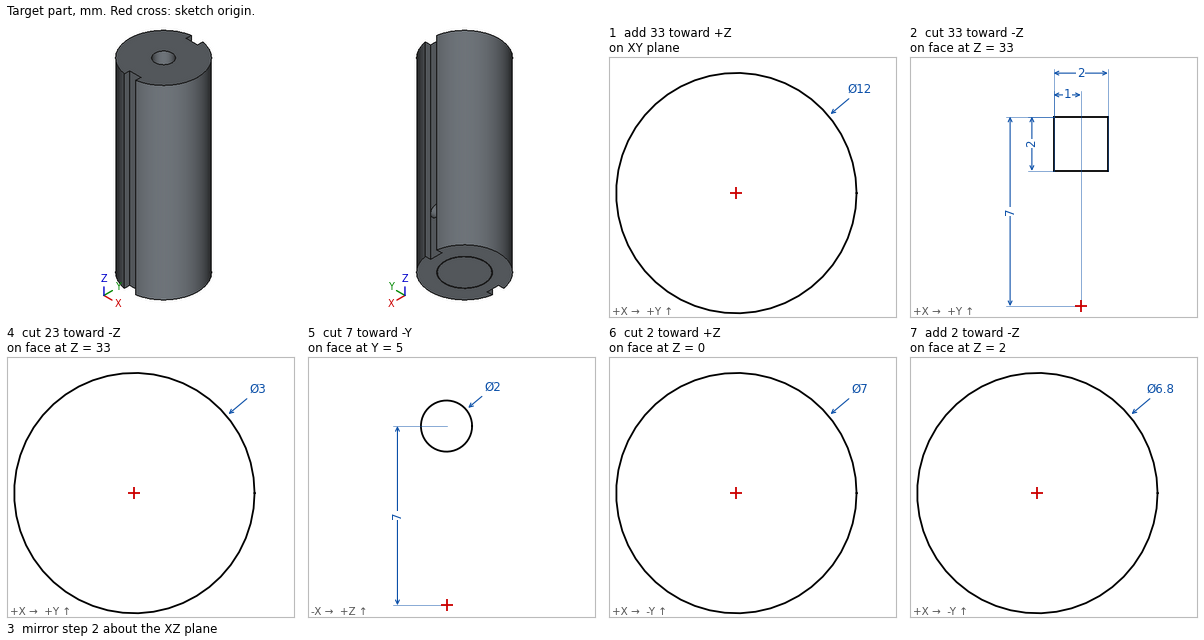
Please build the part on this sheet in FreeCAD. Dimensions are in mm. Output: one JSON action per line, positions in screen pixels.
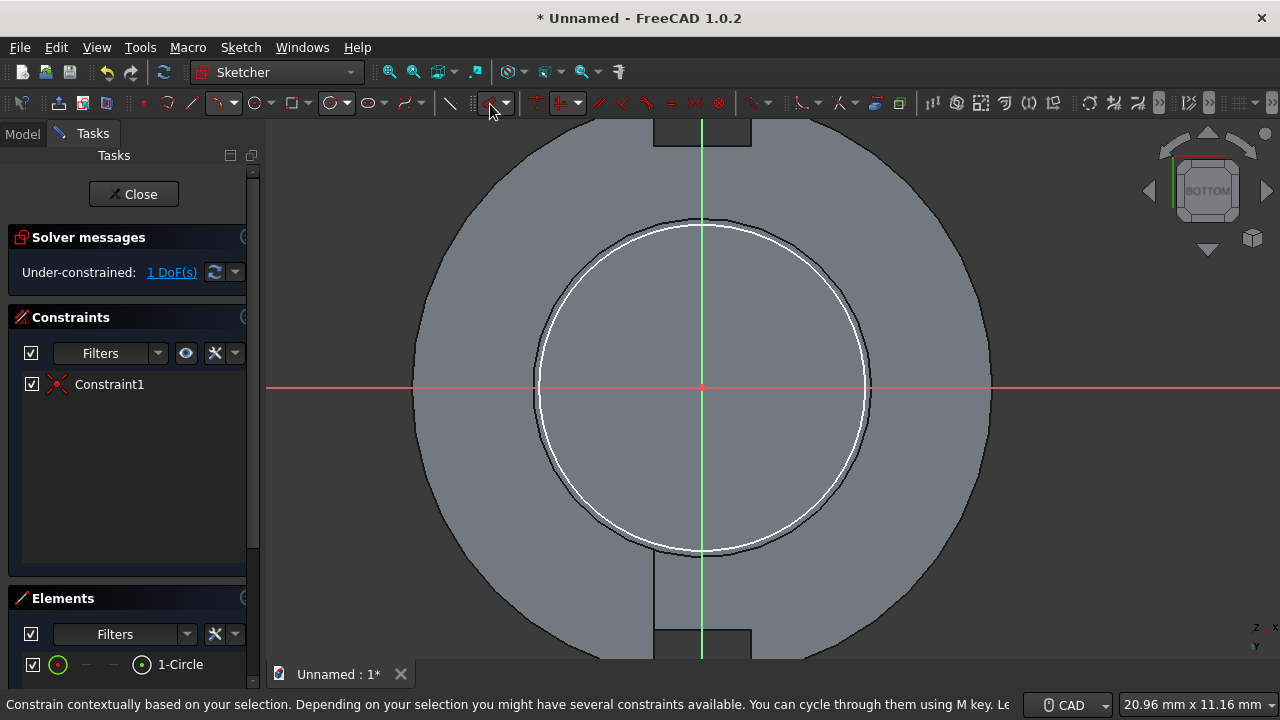
{"action": "left_click", "coordinate": [817, 272]}
{"action": "left_click", "coordinate": [840, 249]}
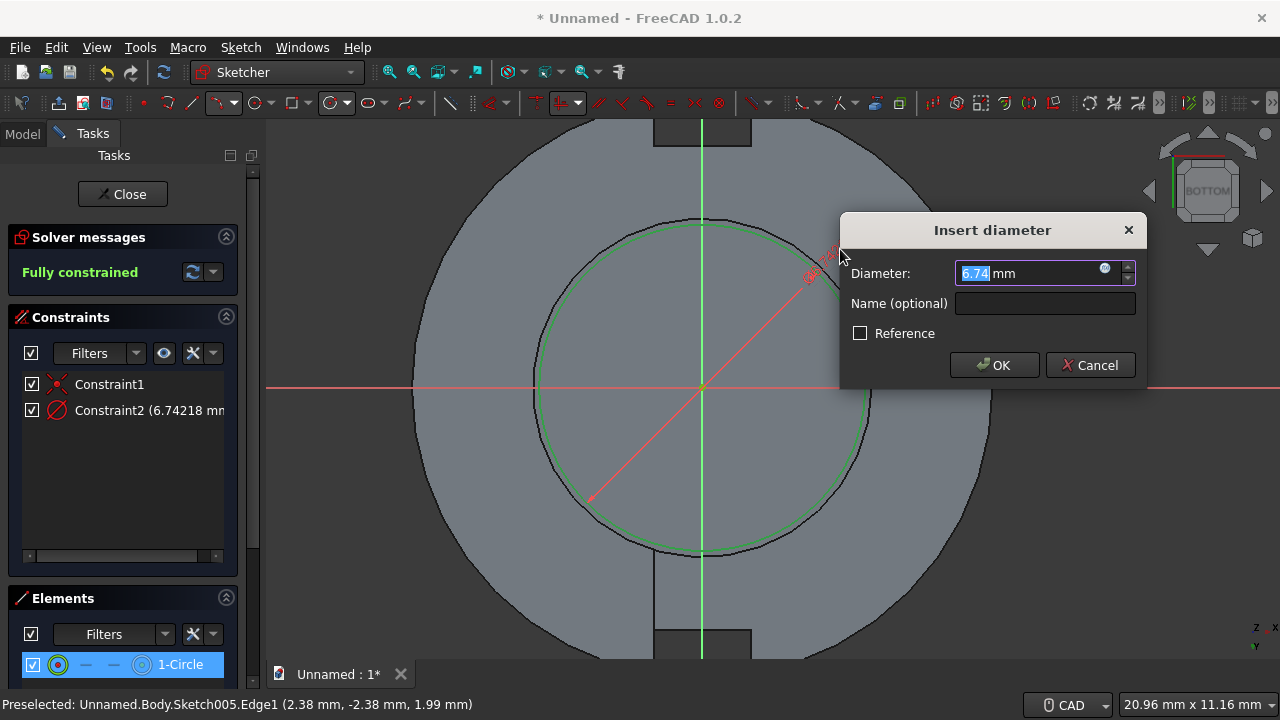
{"action": "type", "text": "6.8"}
{"action": "key", "text": "Return"}
{"action": "key", "text": "Escape"}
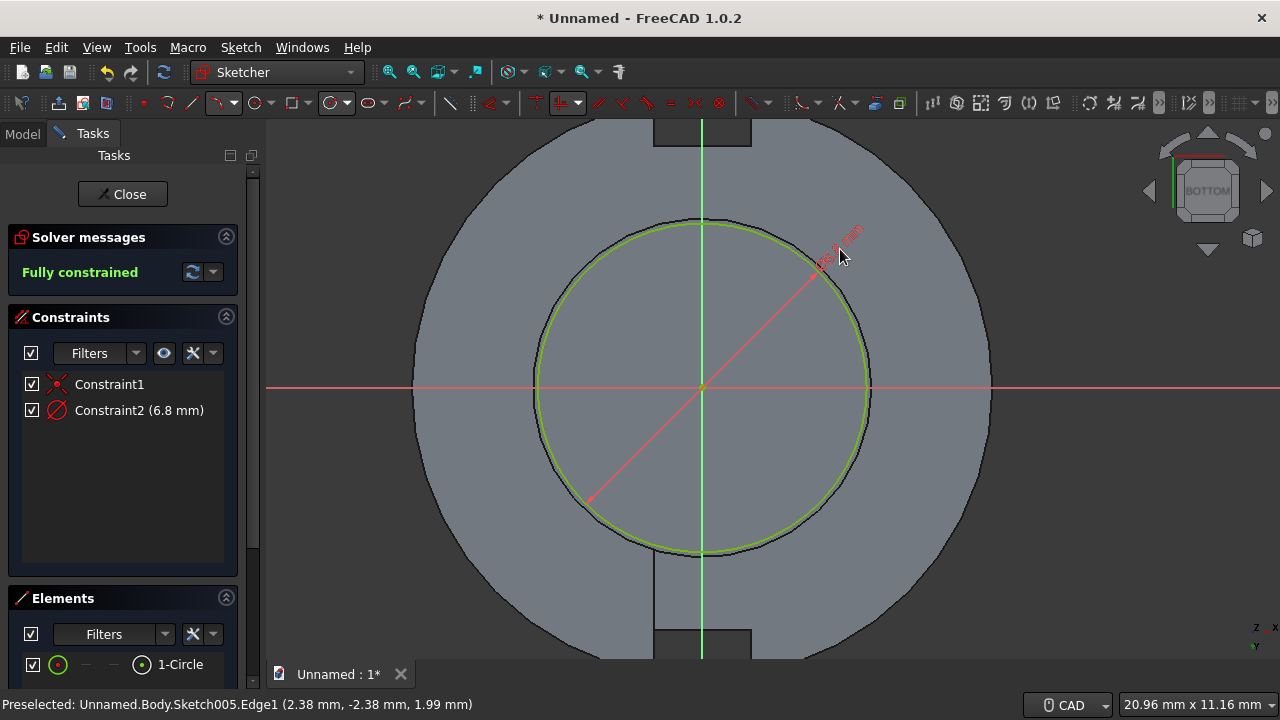
{"action": "left_click", "coordinate": [123, 194]}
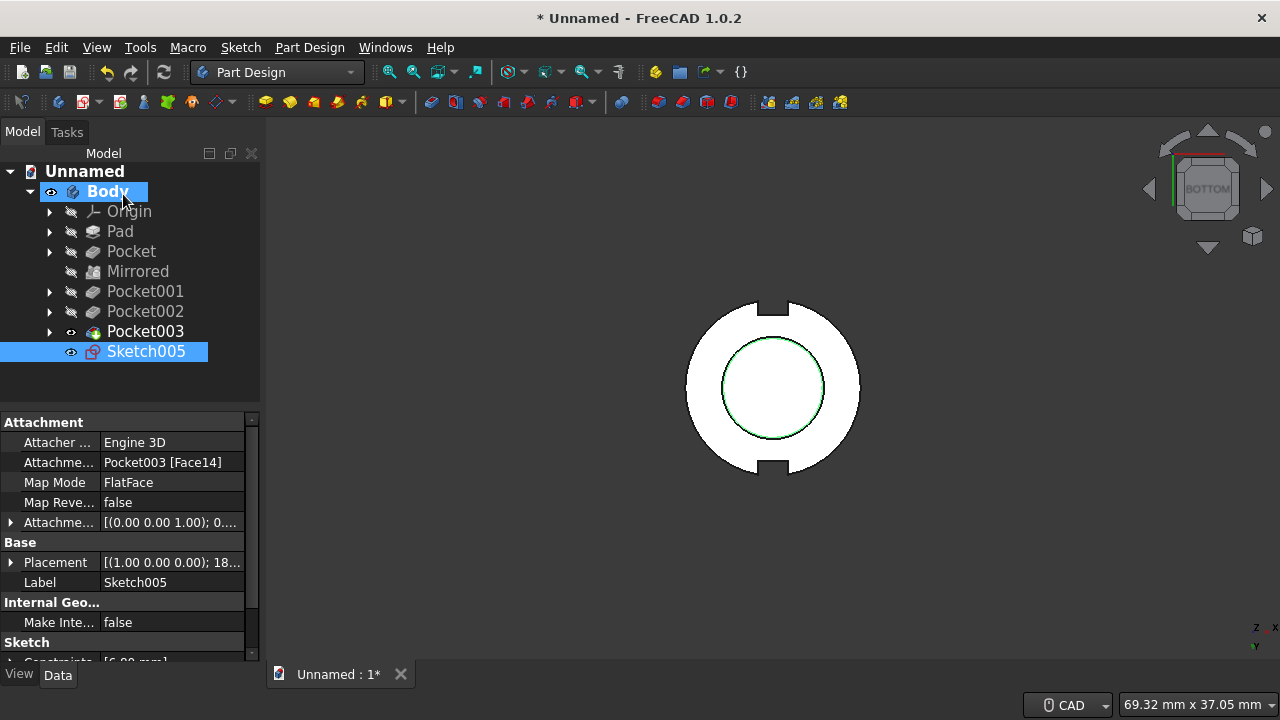
{"action": "left_click", "coordinate": [266, 102]}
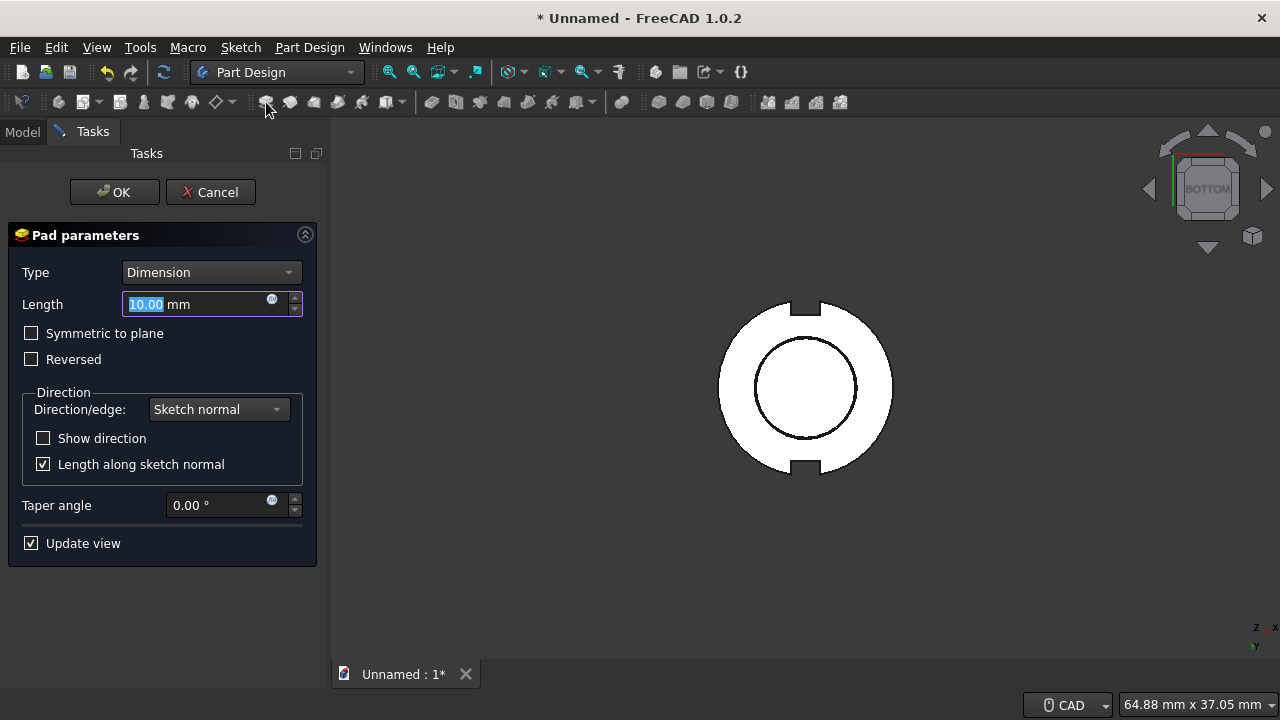
{"action": "type", "text": "2"}
{"action": "key", "text": "Tab"}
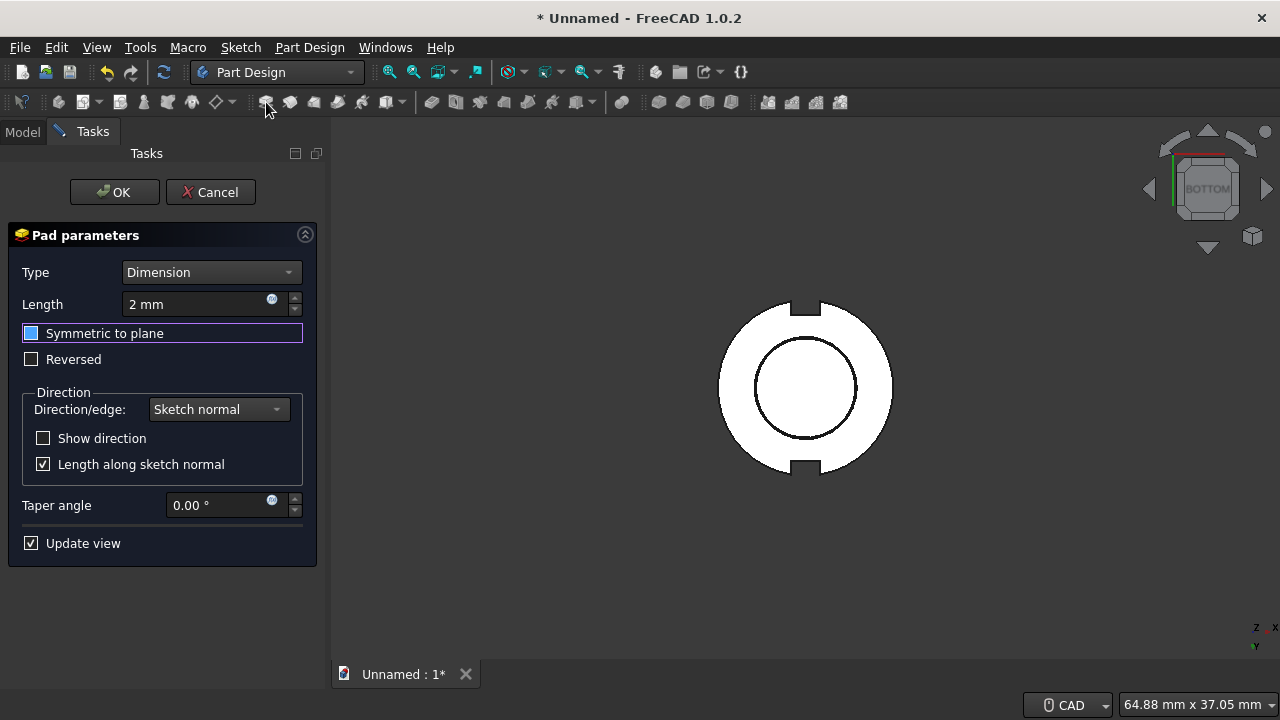
{"action": "left_click", "coordinate": [115, 192]}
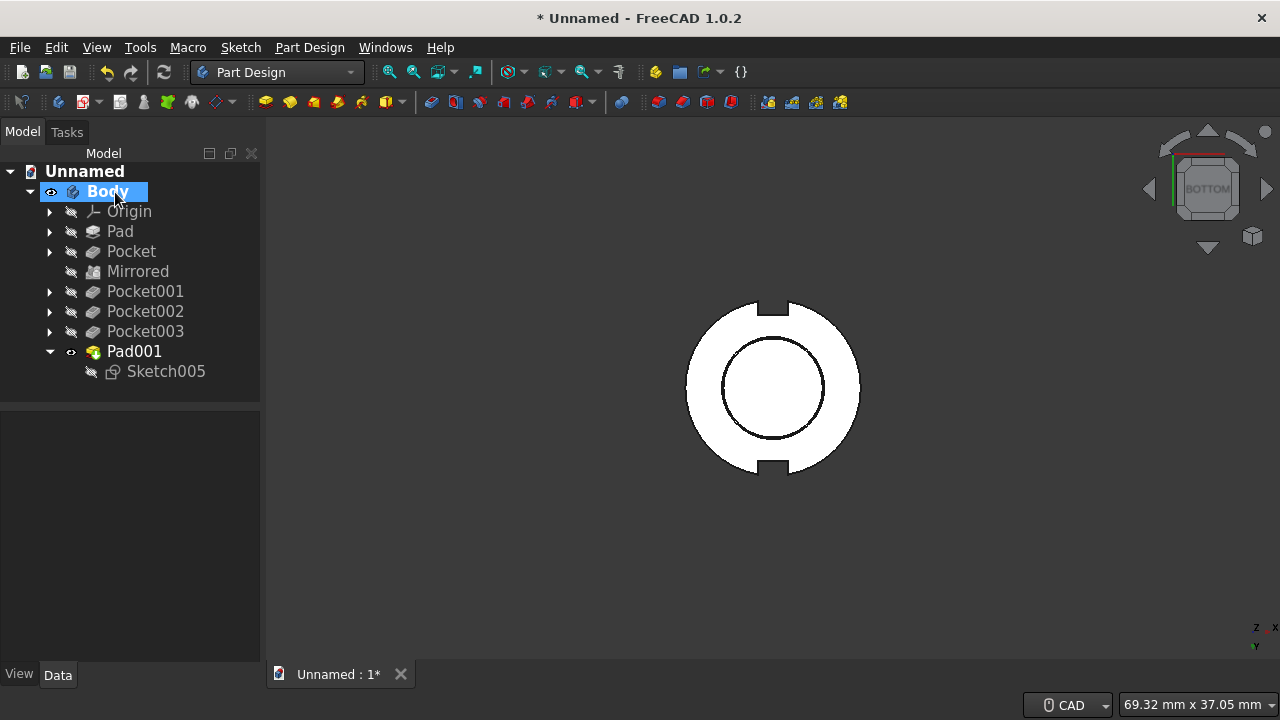
{"action": "key", "text": "0"}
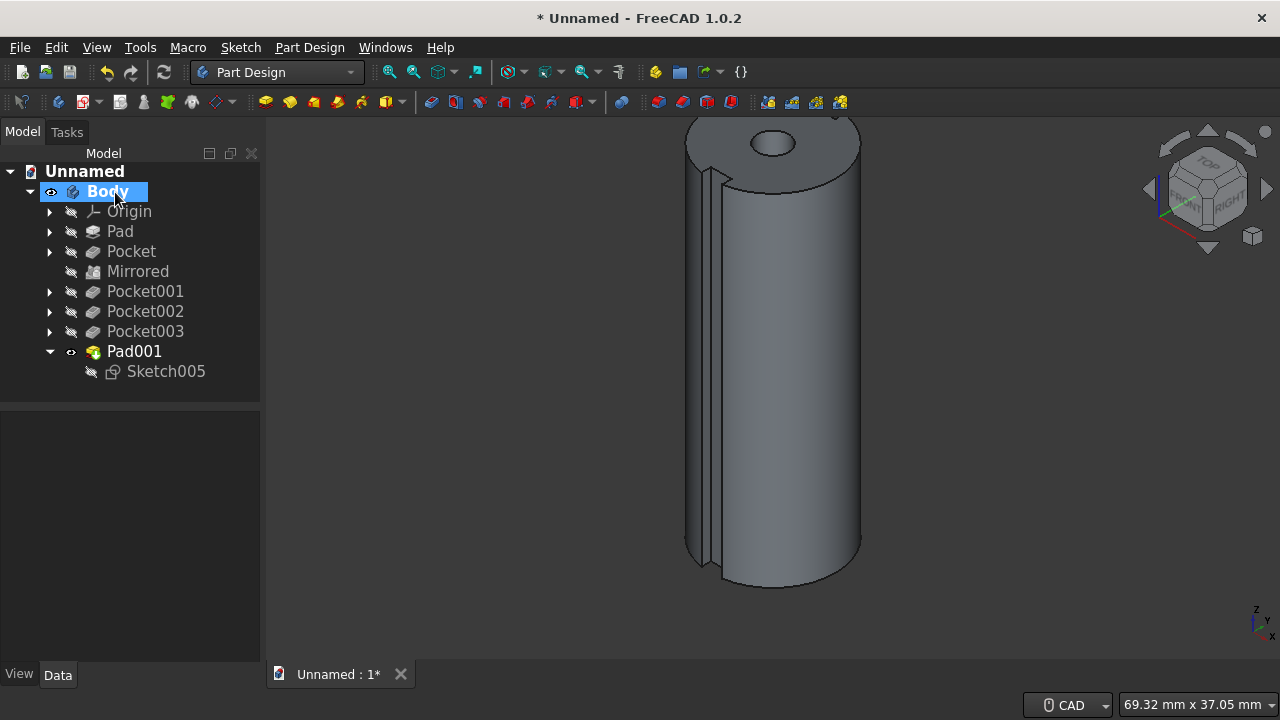
{"action": "key", "text": "v f"}